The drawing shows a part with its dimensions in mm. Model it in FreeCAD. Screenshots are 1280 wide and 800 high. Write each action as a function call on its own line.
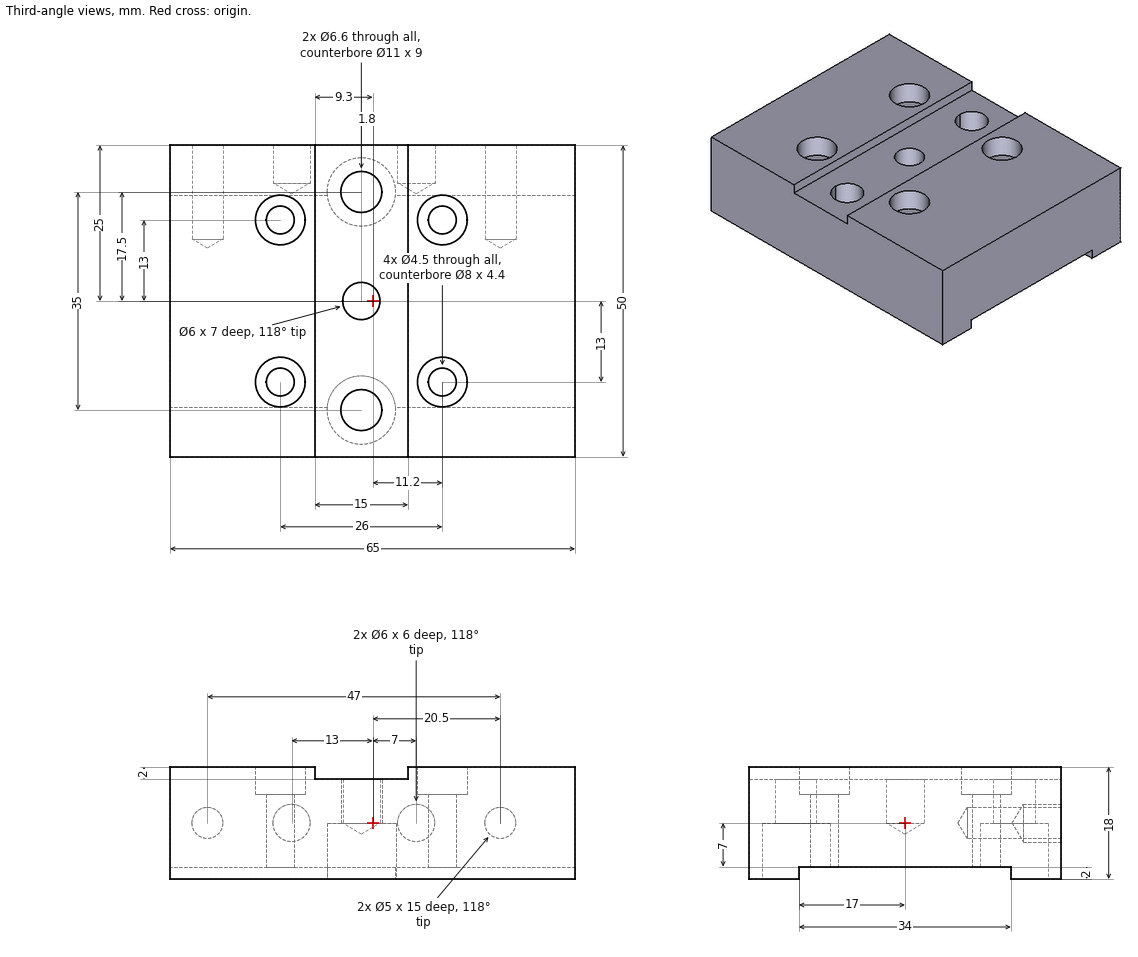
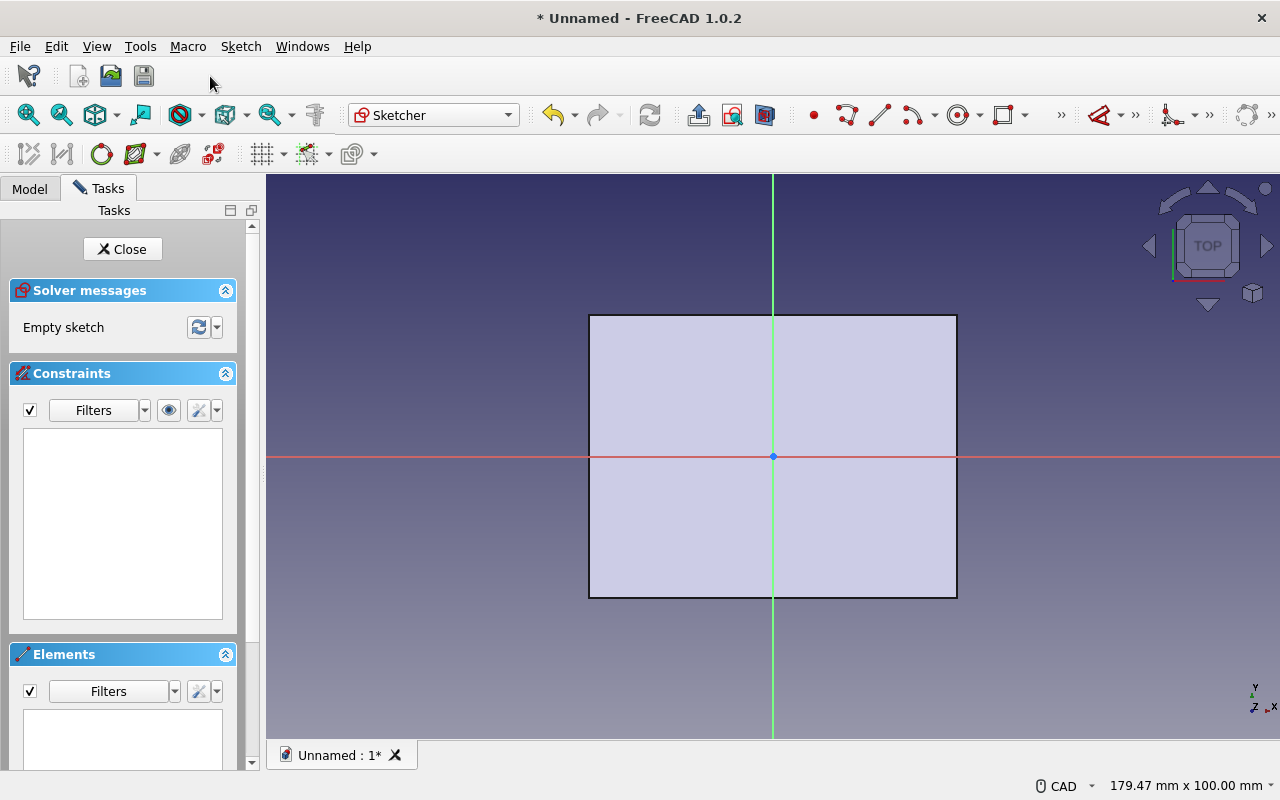
scroll(810, 456, up, 4)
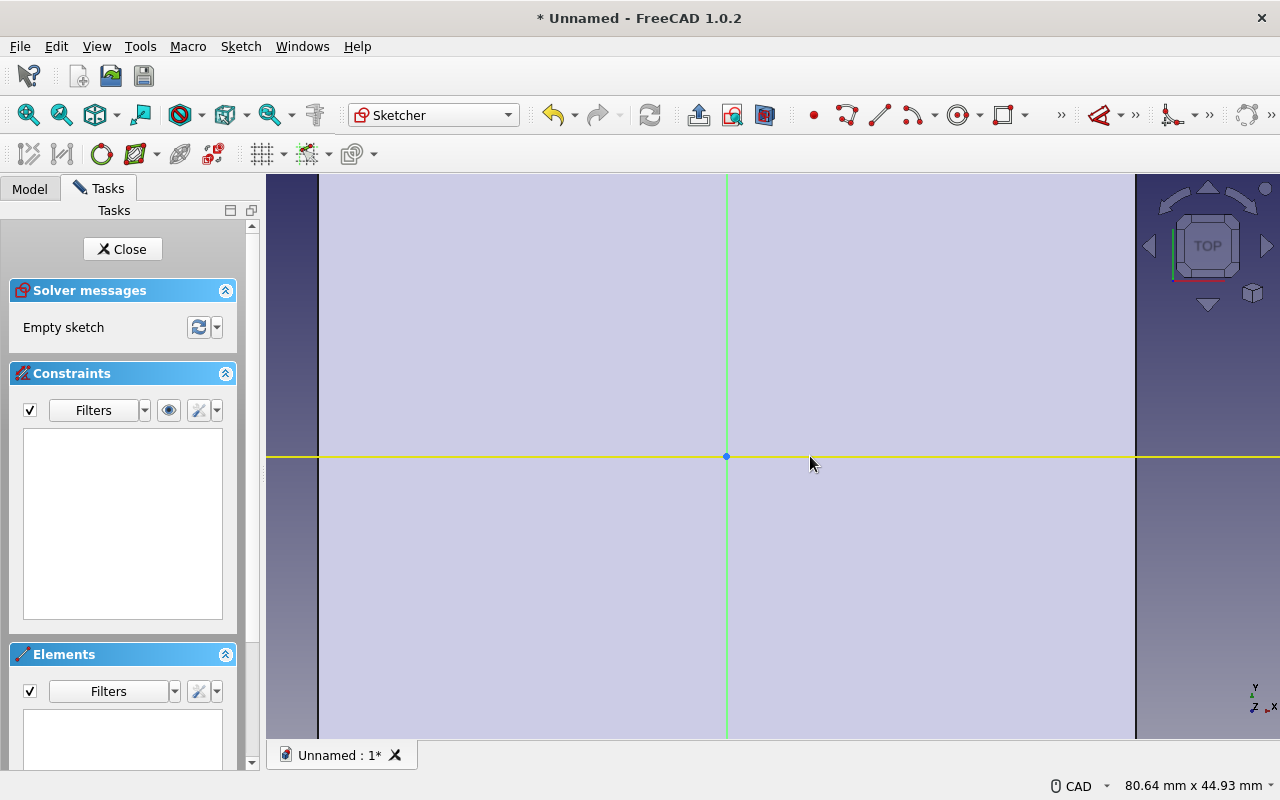
key(g)
key(c)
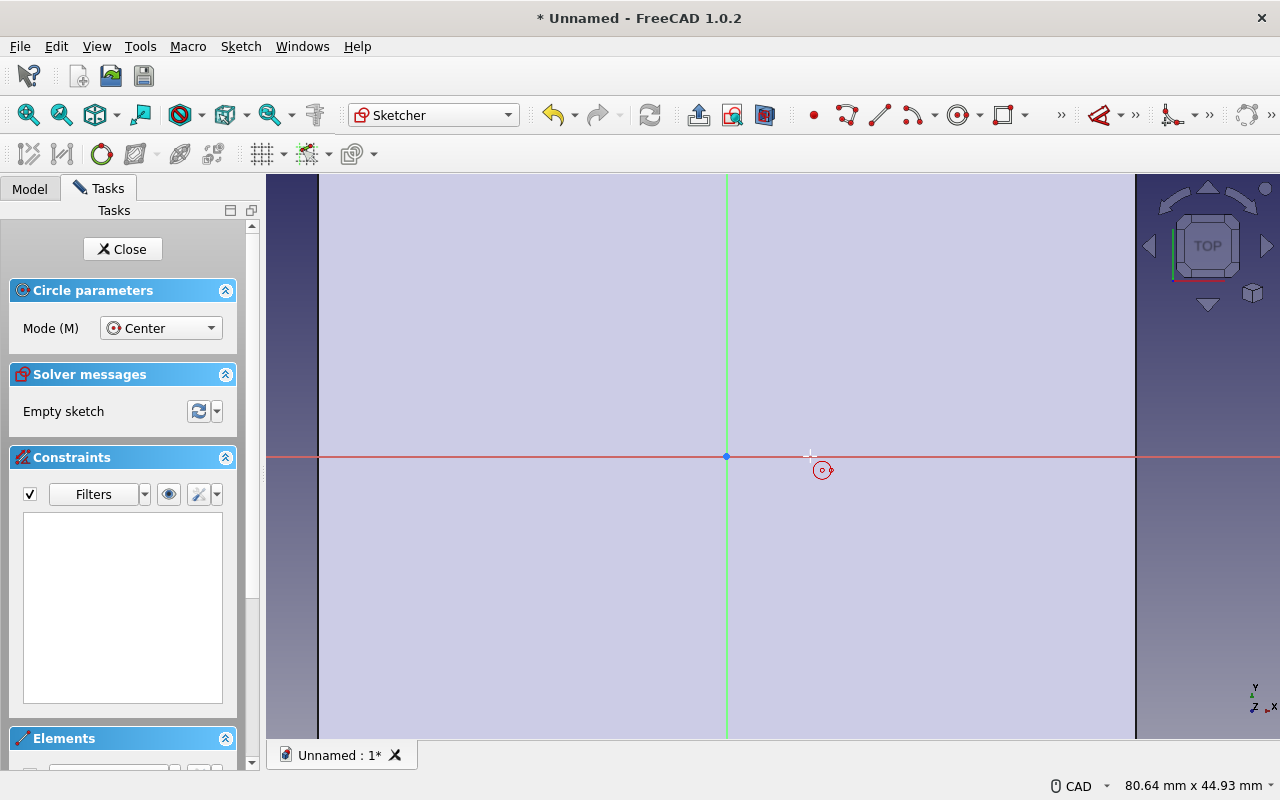
click(868, 620)
move(888, 600)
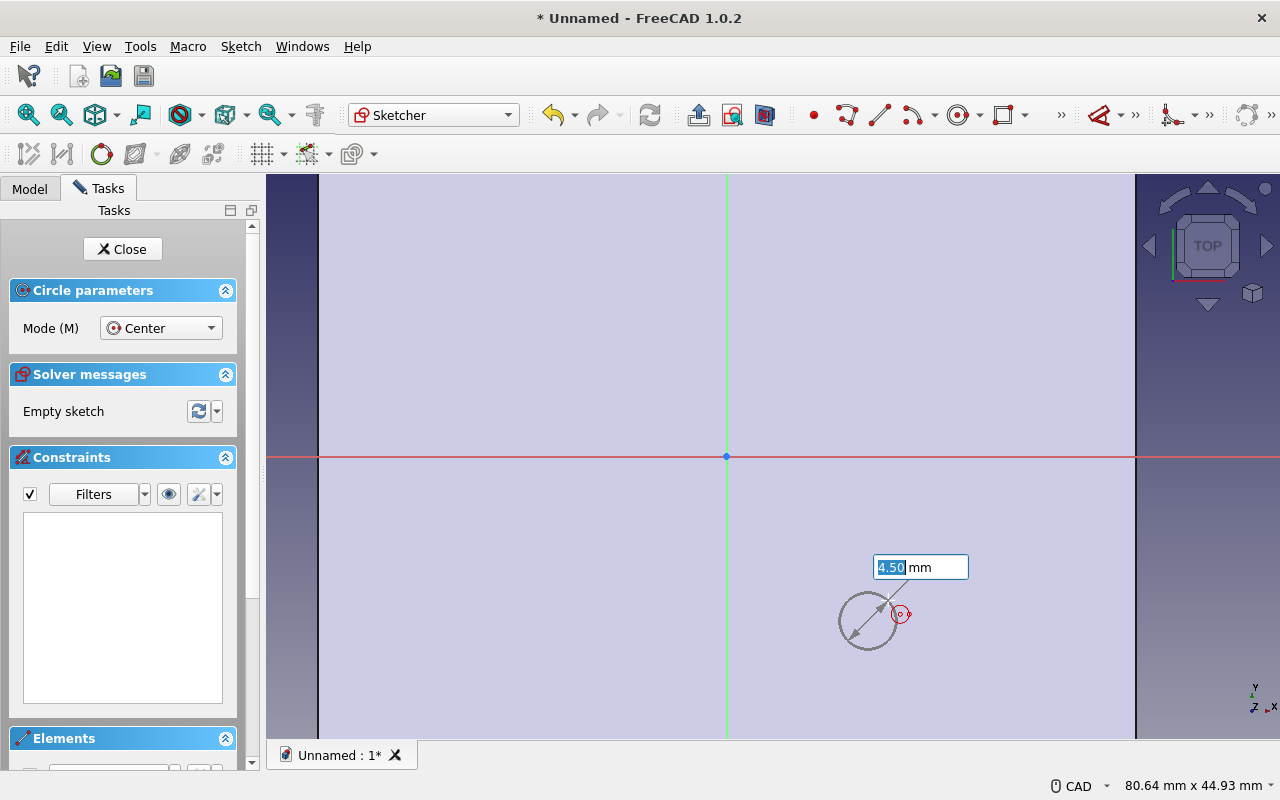
text(4.5)
key(Return)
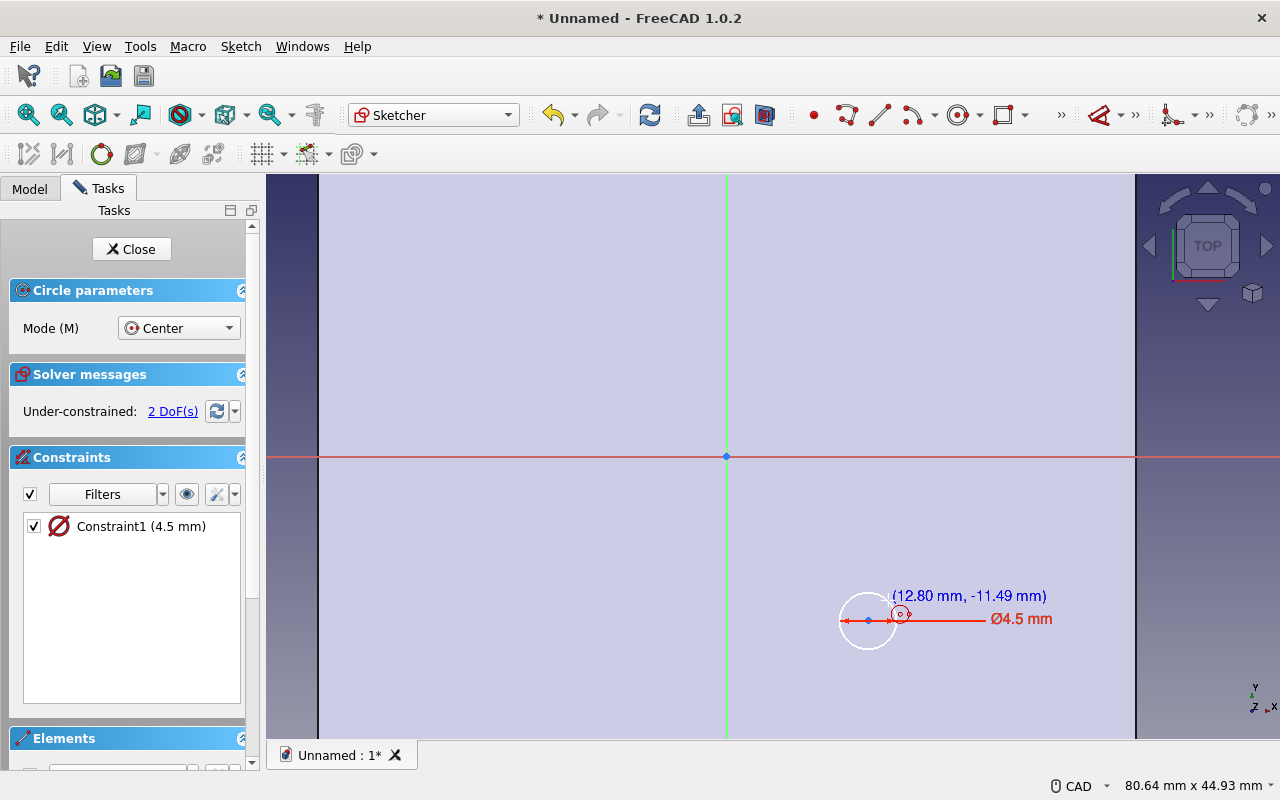
click(541, 620)
move(561, 600)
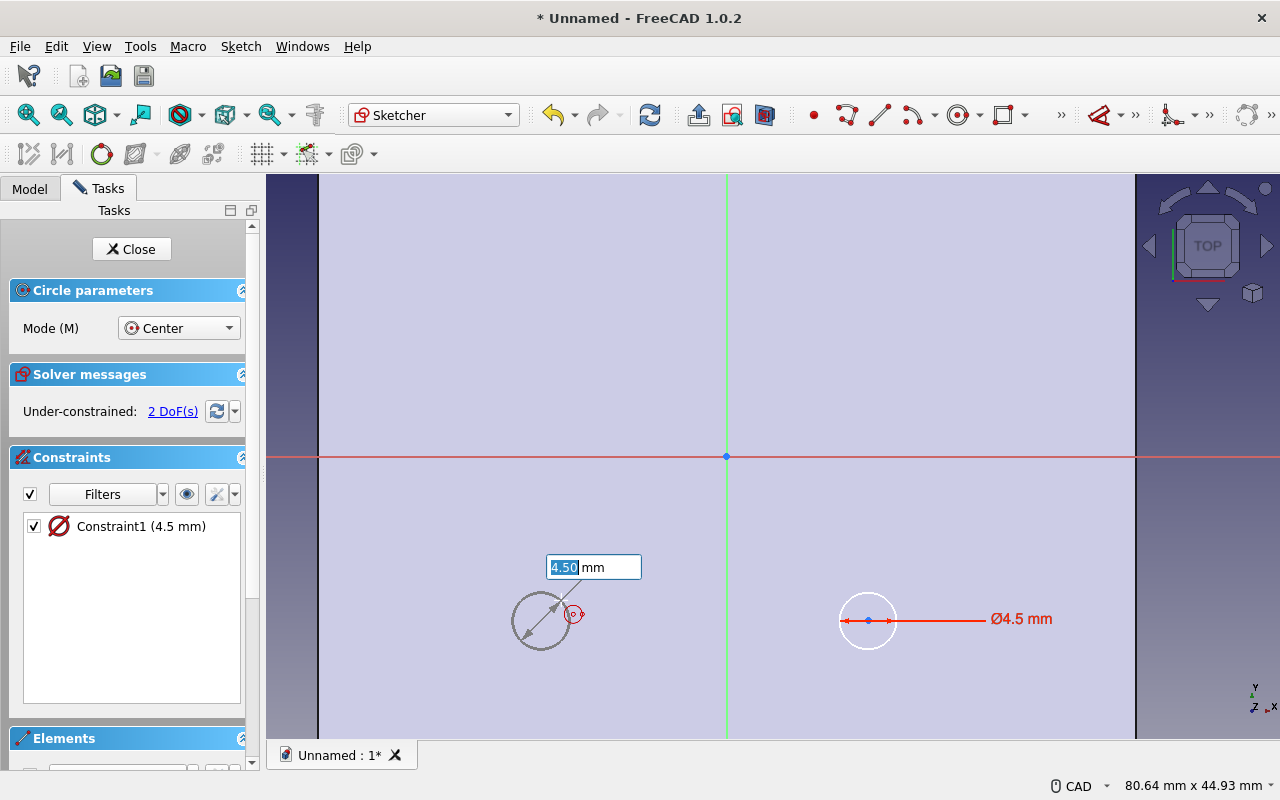
text(4.5)
key(Return)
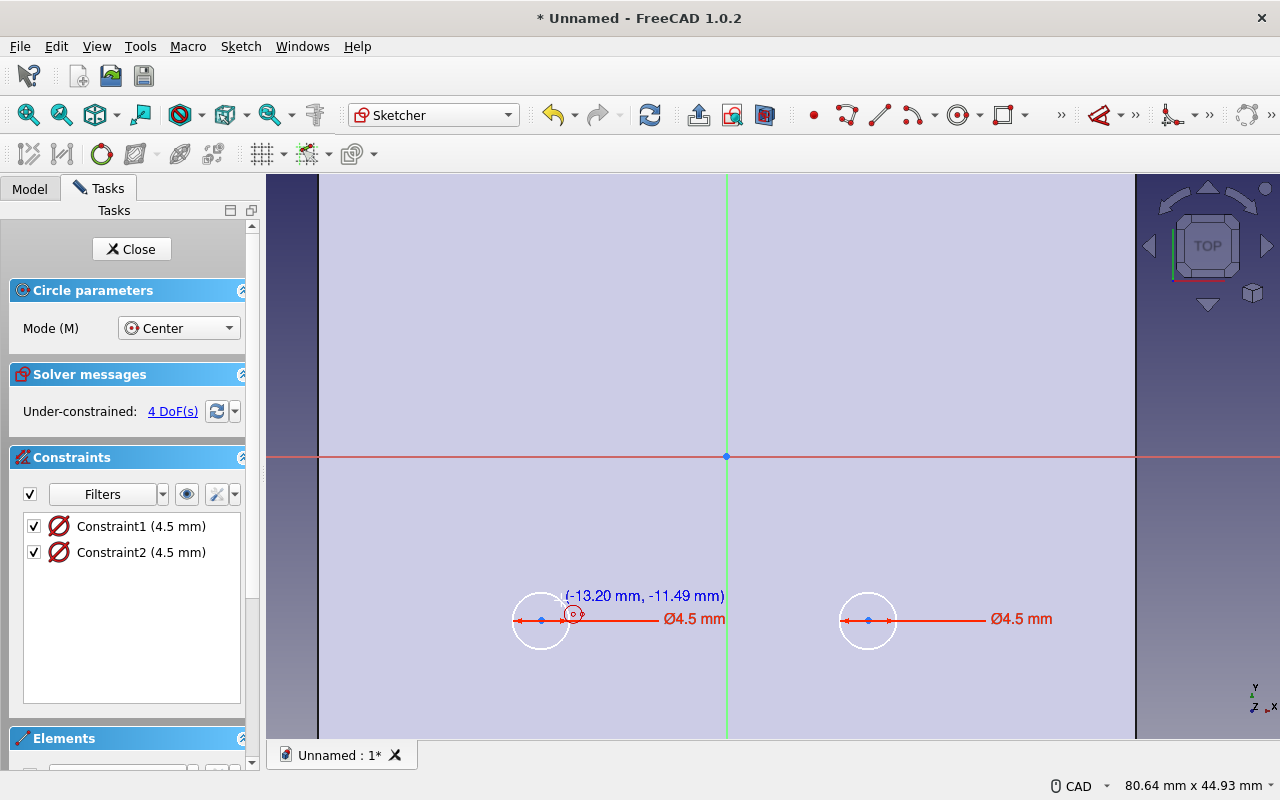
click(541, 293)
move(561, 273)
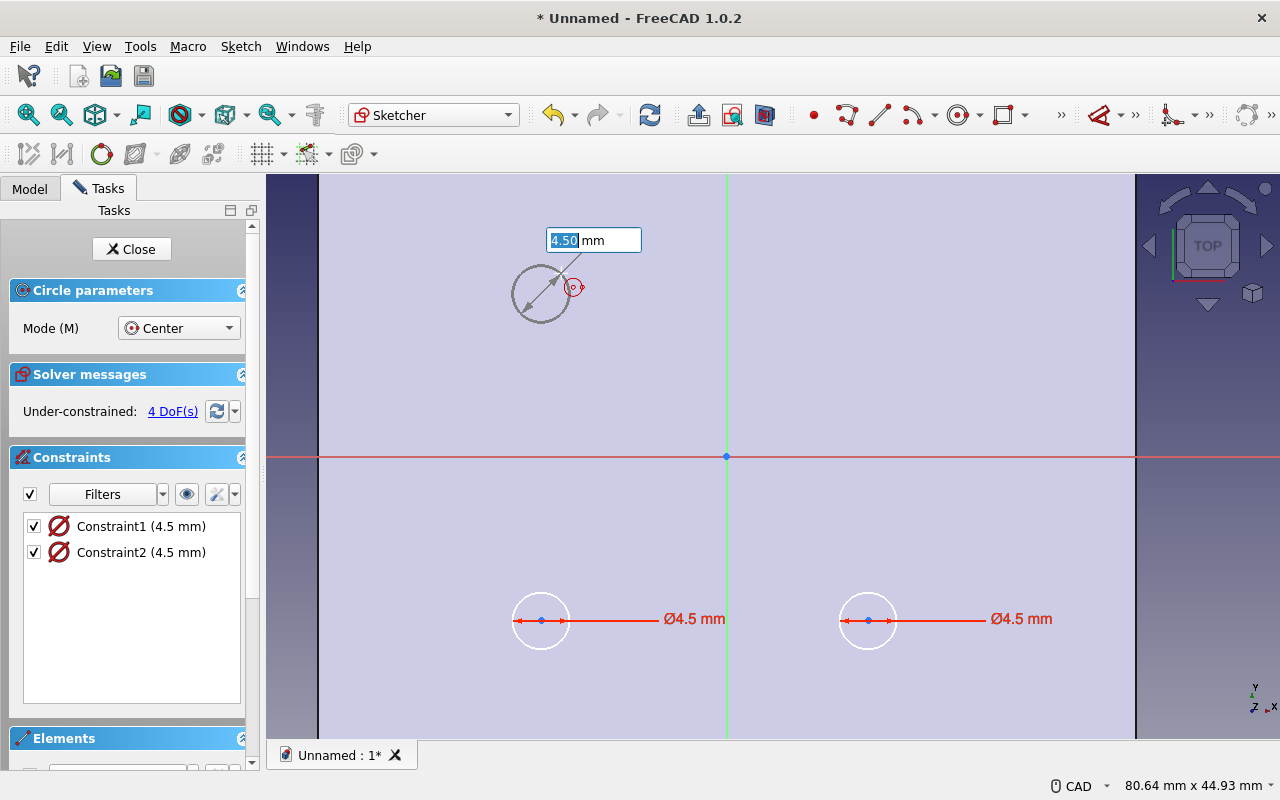
text(4.5)
key(Return)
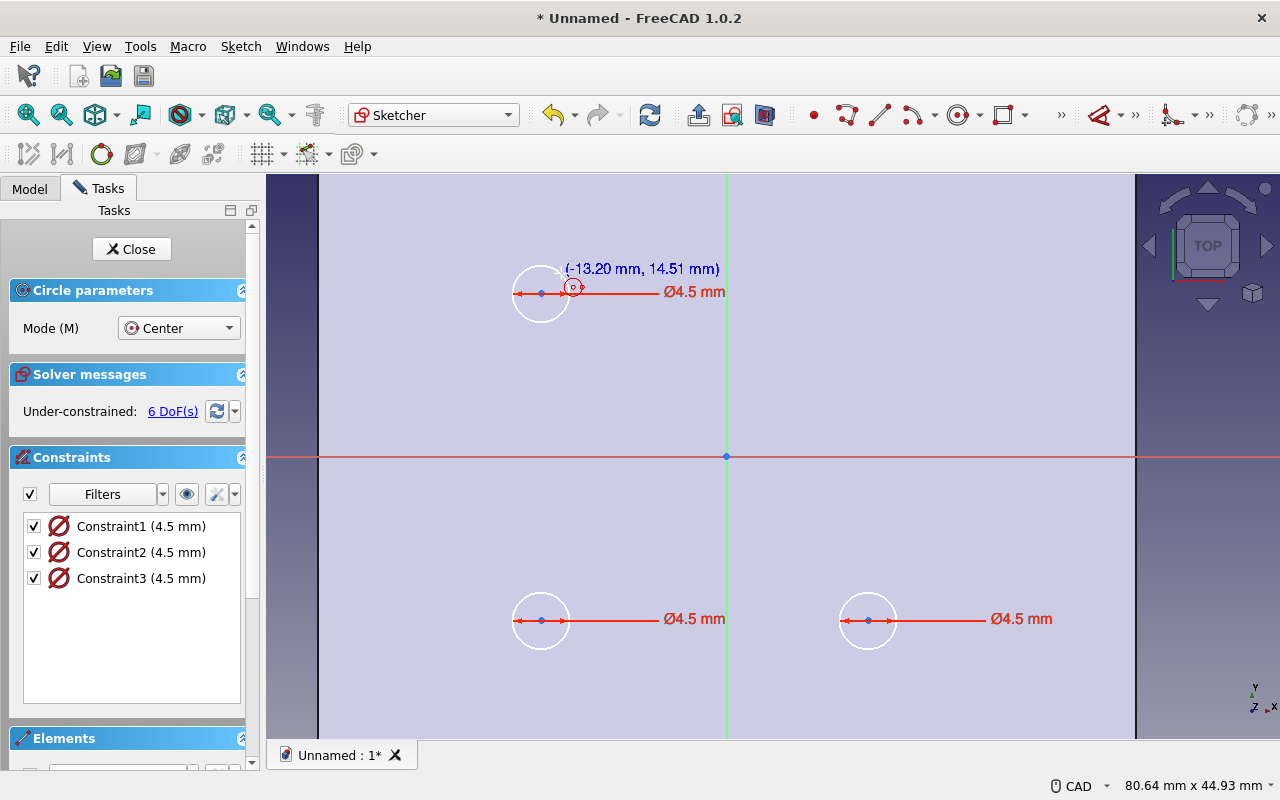
click(868, 293)
move(888, 273)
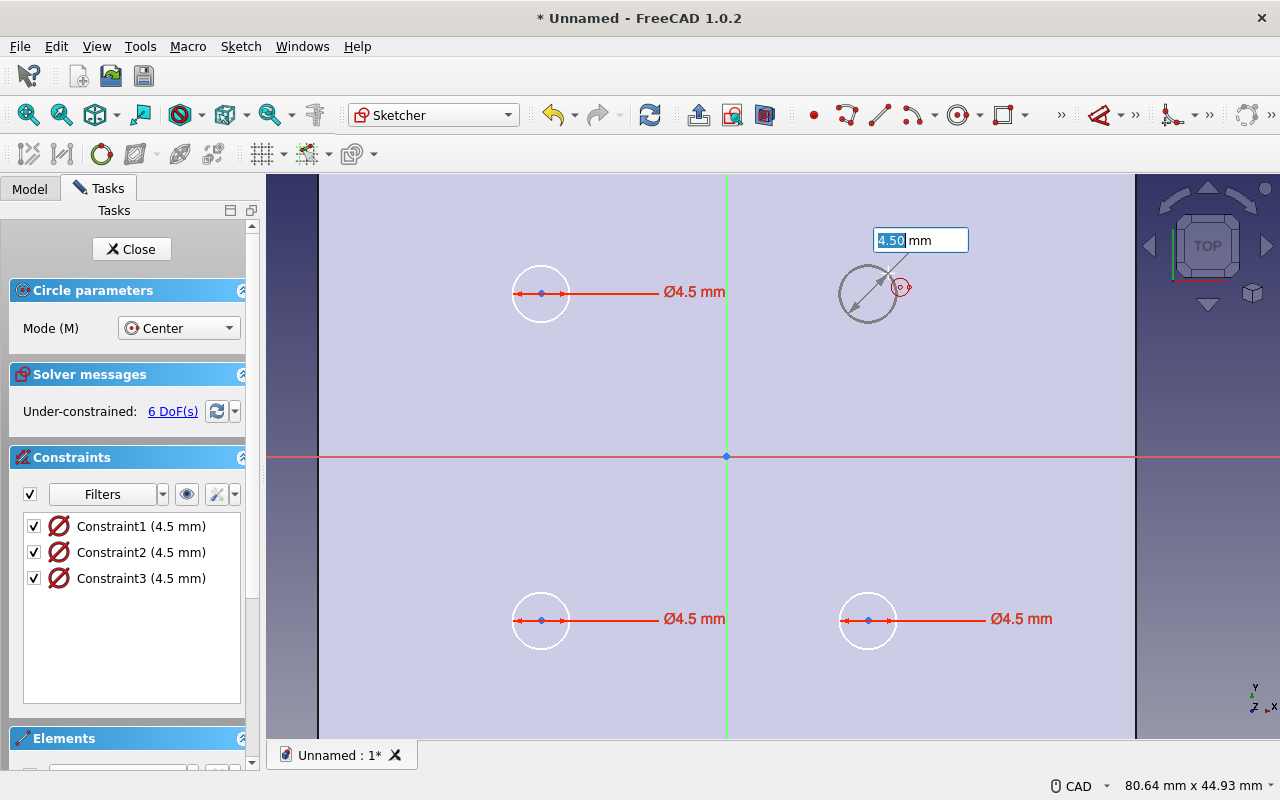
text(4.5)
key(Return)
key(Escape)